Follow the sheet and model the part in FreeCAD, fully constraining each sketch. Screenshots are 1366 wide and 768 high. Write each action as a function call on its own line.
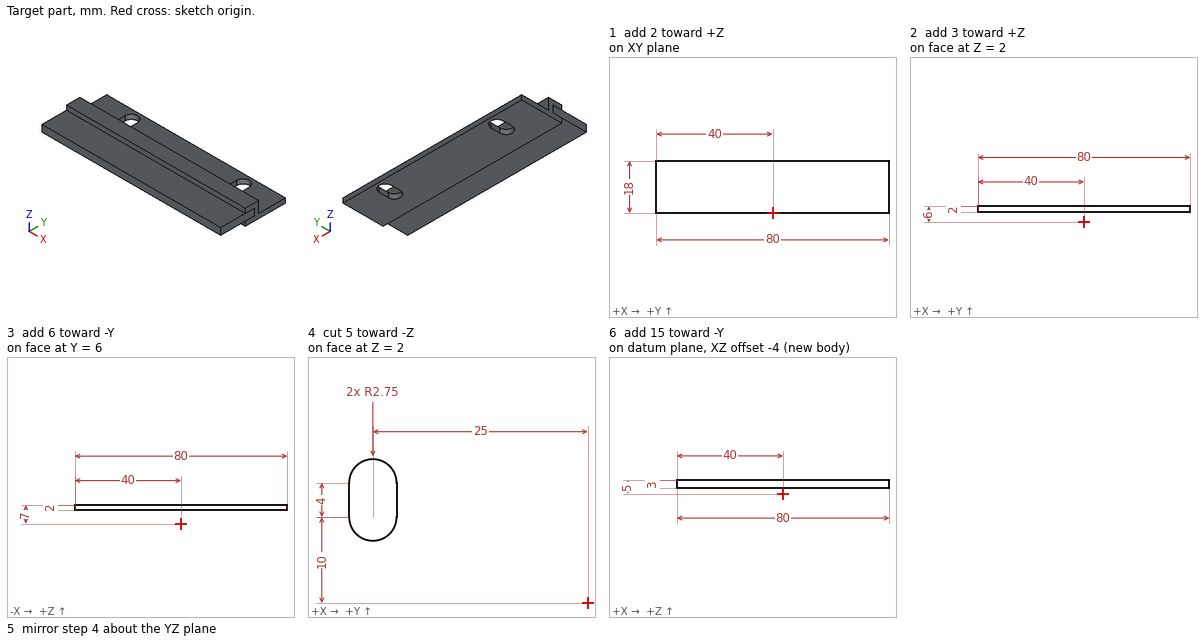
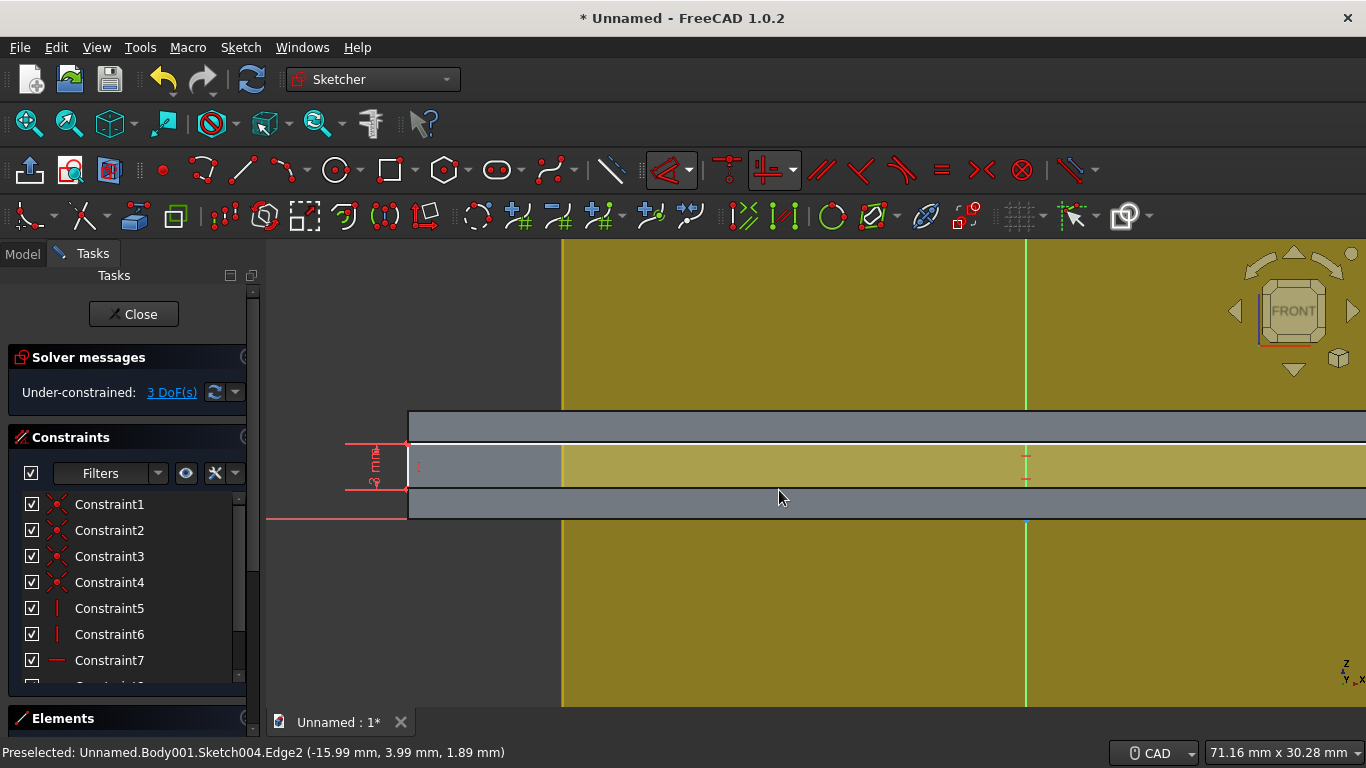
key(l)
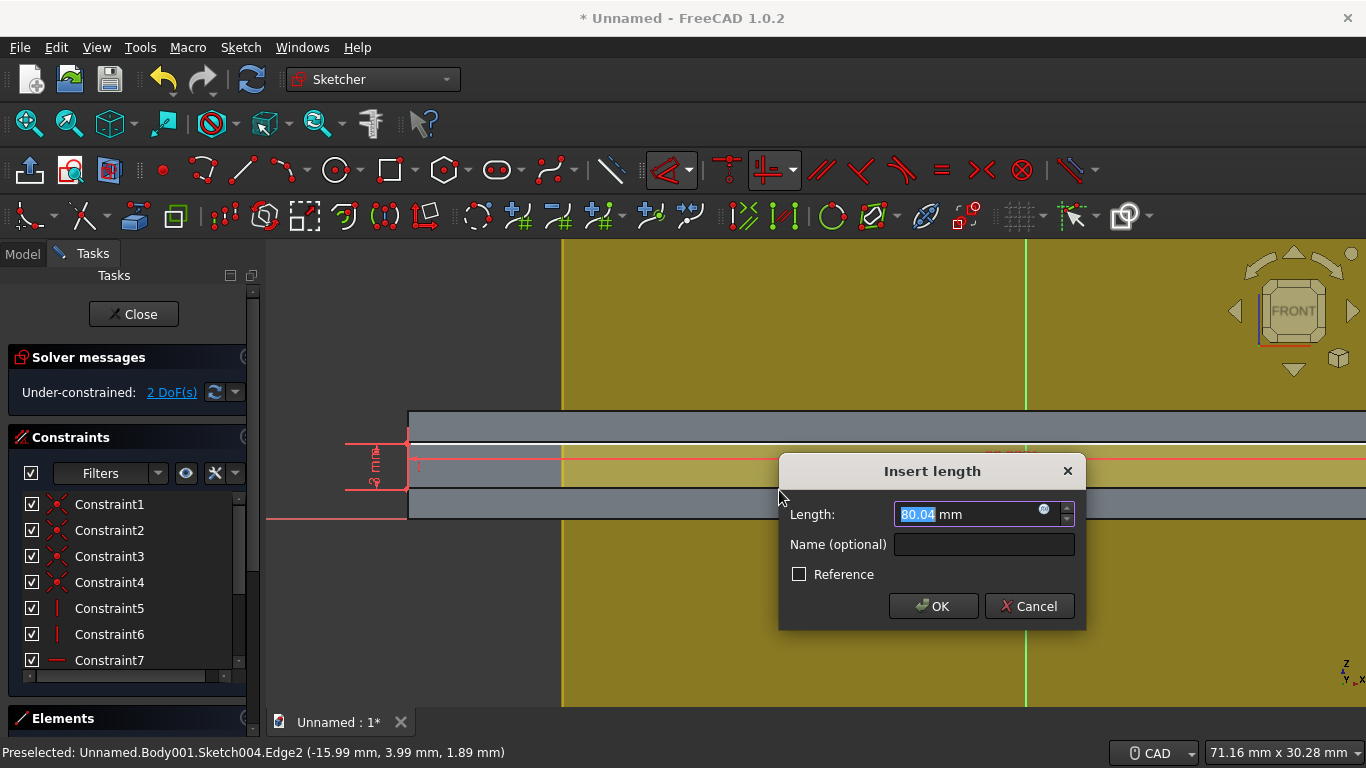
text(80)
key(Return)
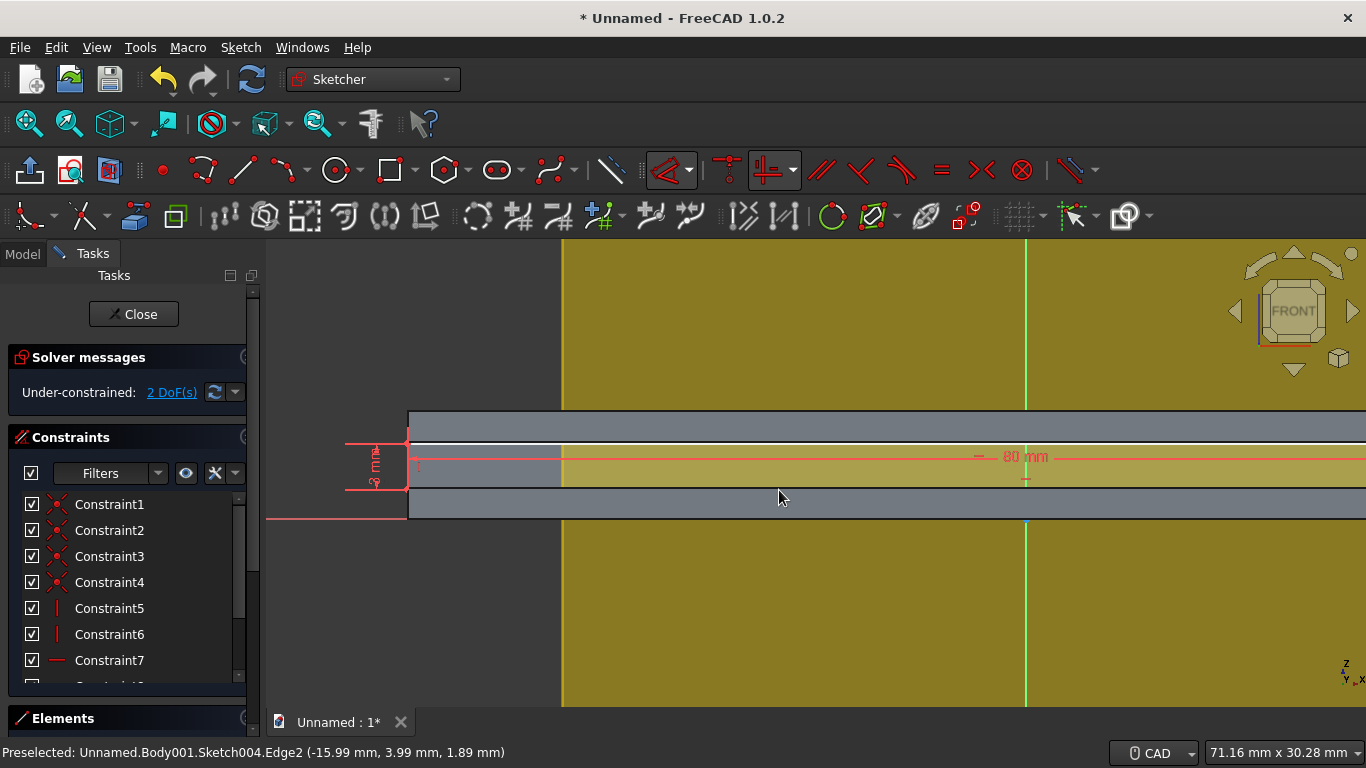
click(408, 444)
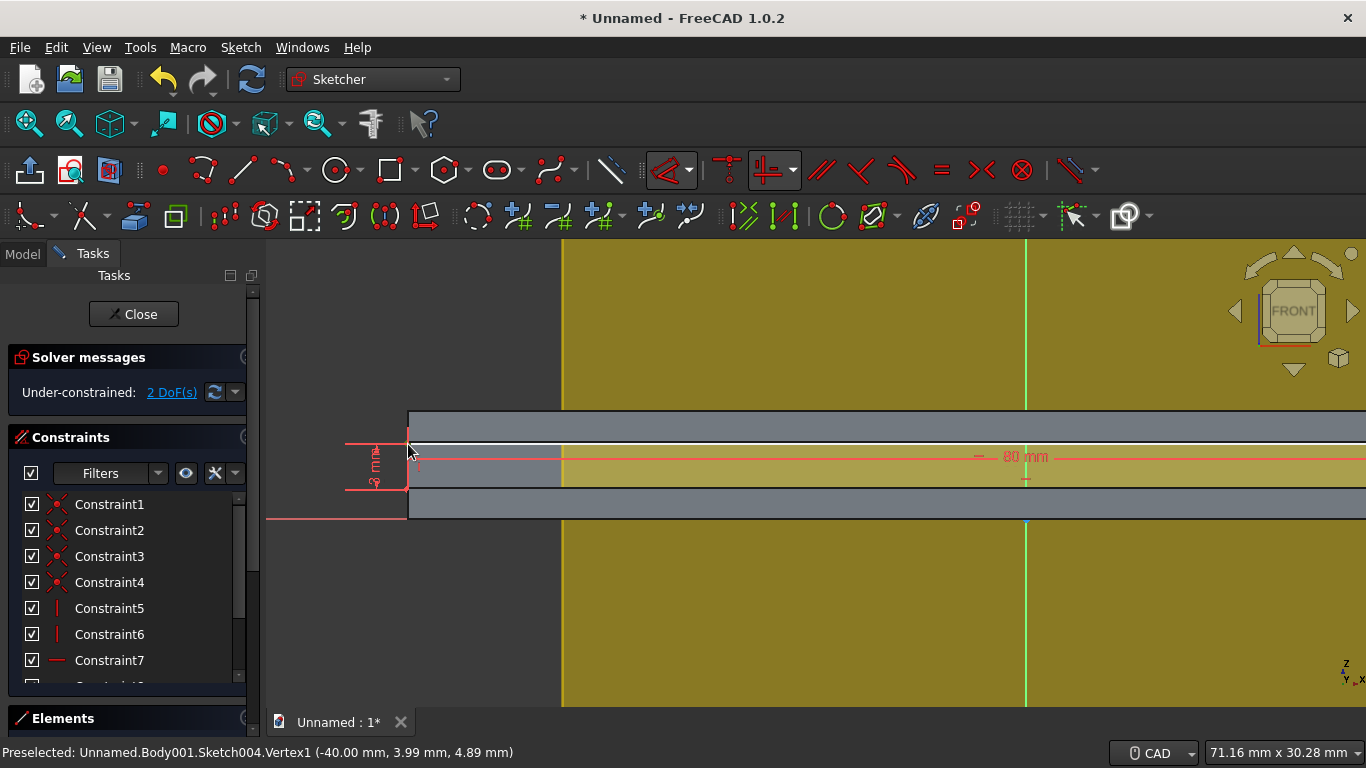
key(i)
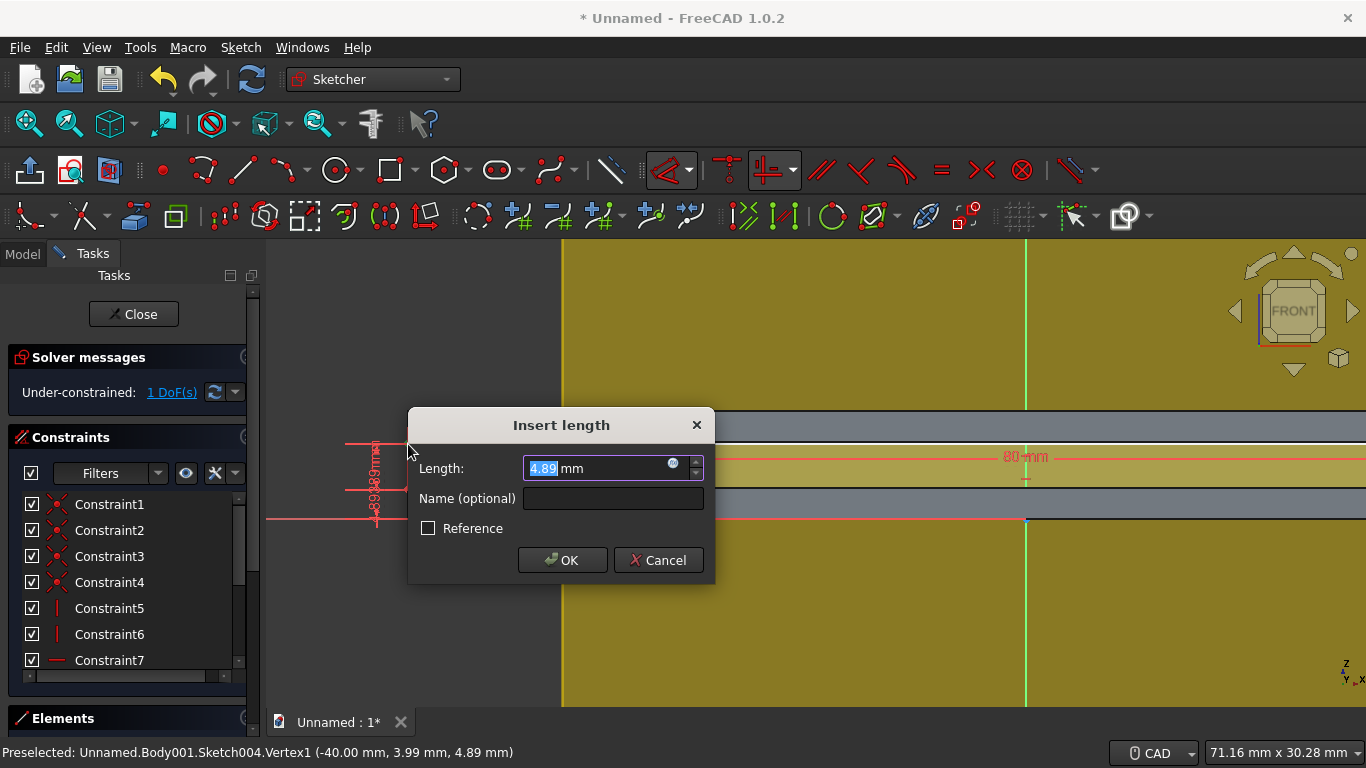
text(5)
key(Return)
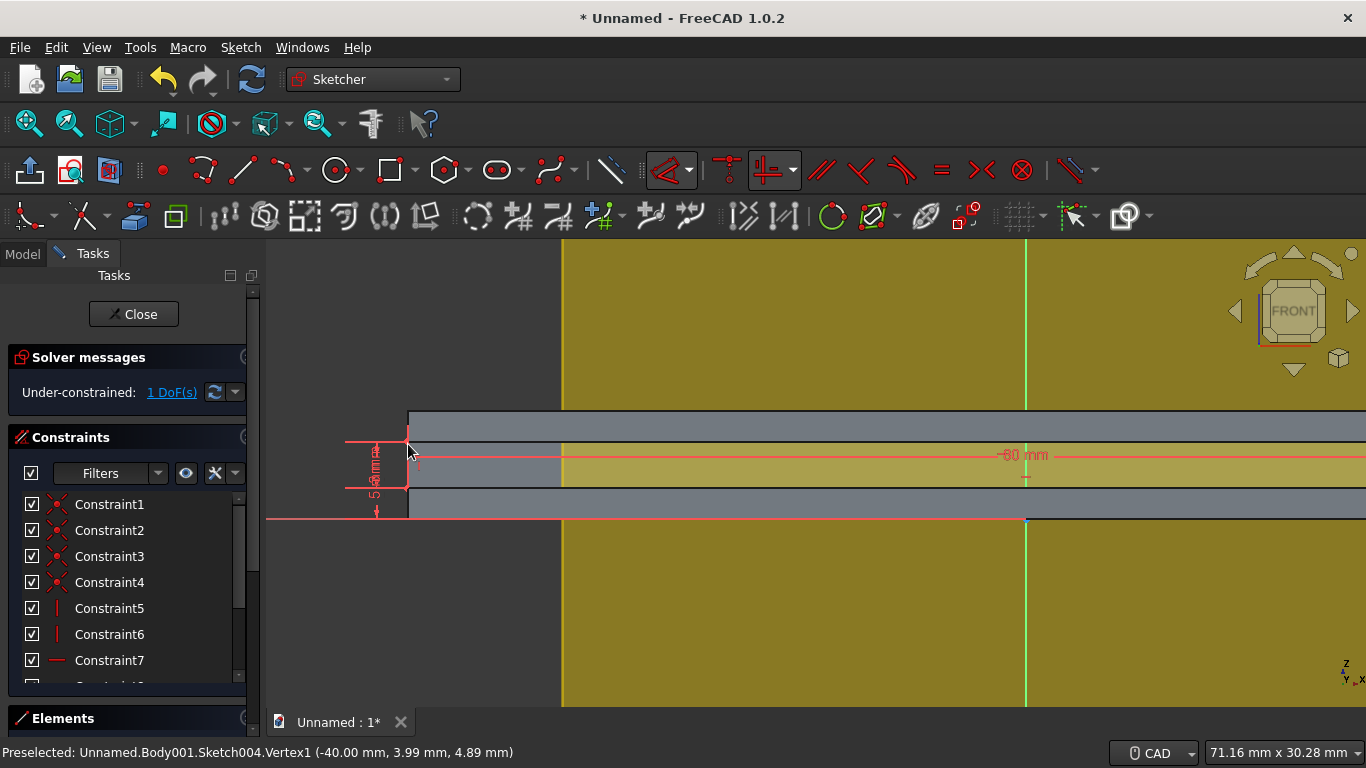
click(408, 442)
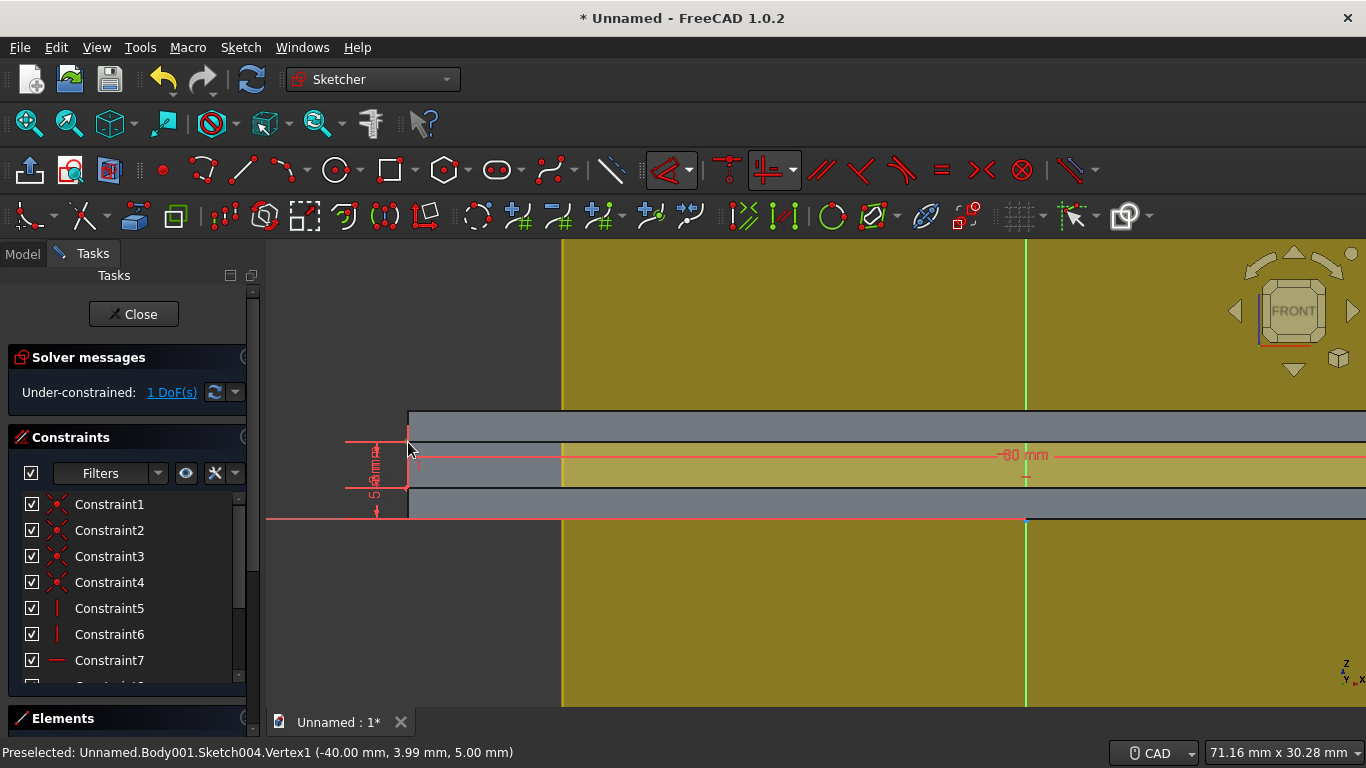
click(692, 170)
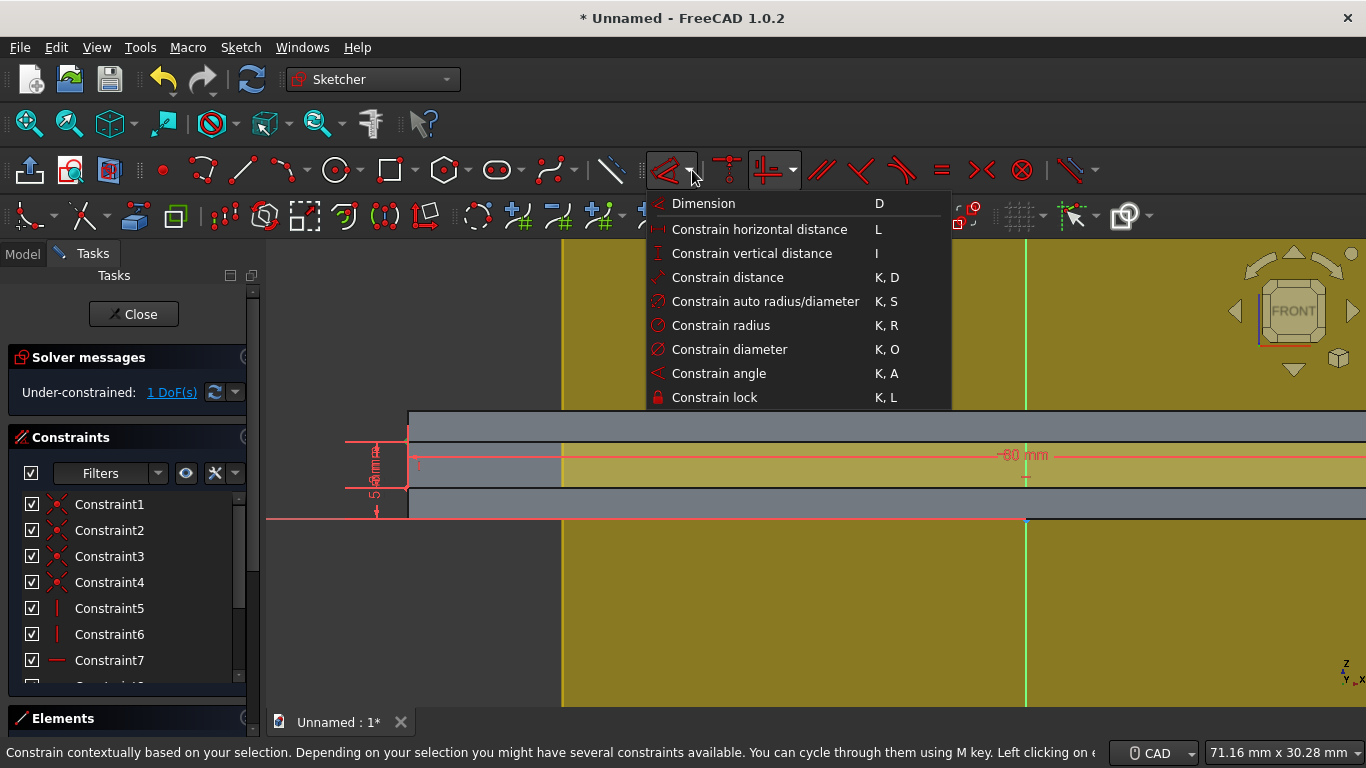
click(799, 229)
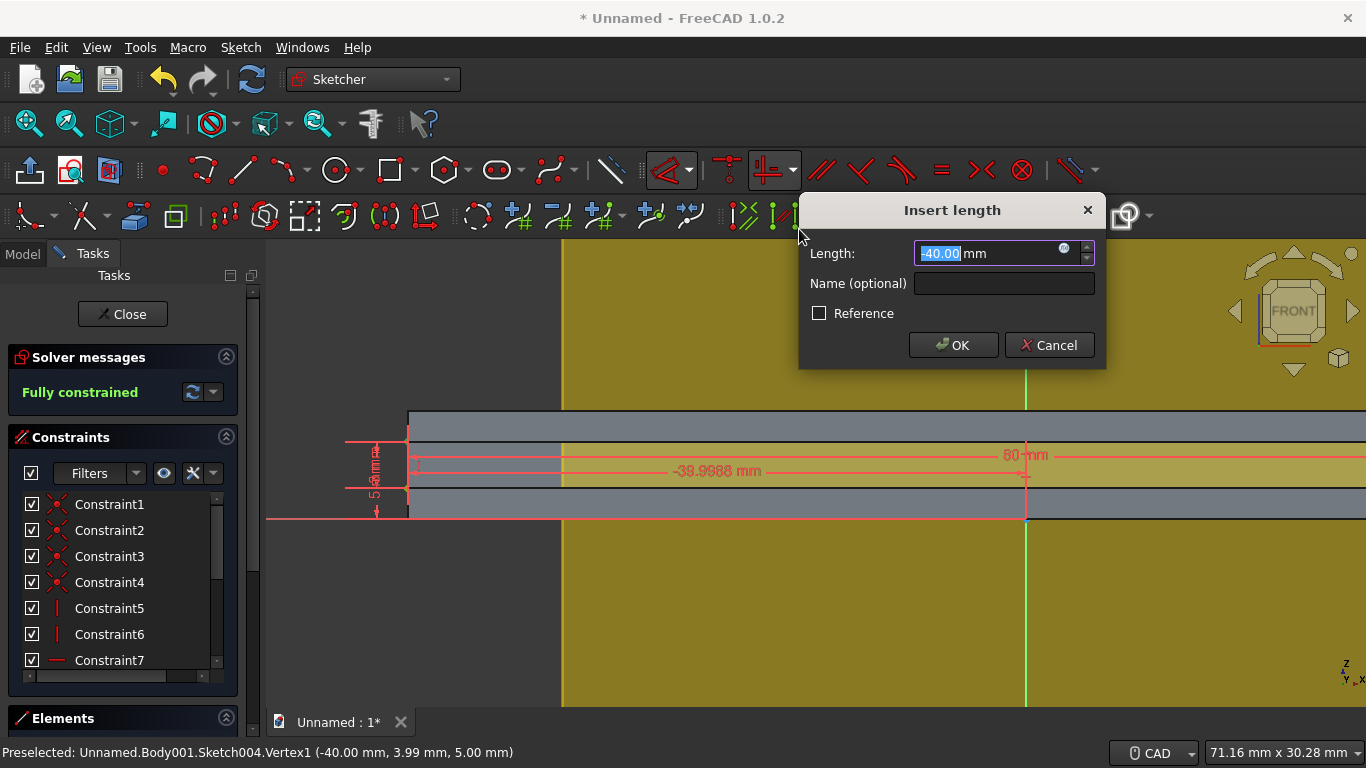
text(-40)
key(Return)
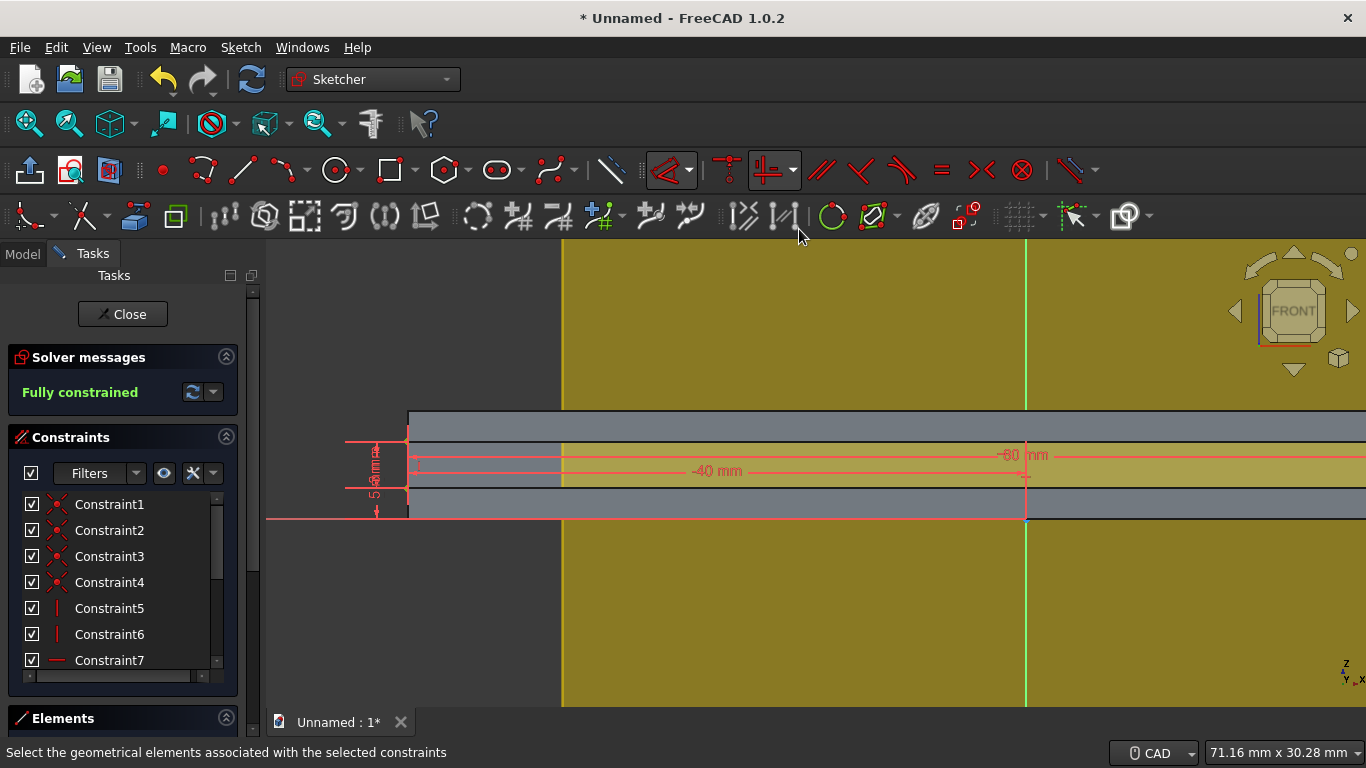
click(123, 314)